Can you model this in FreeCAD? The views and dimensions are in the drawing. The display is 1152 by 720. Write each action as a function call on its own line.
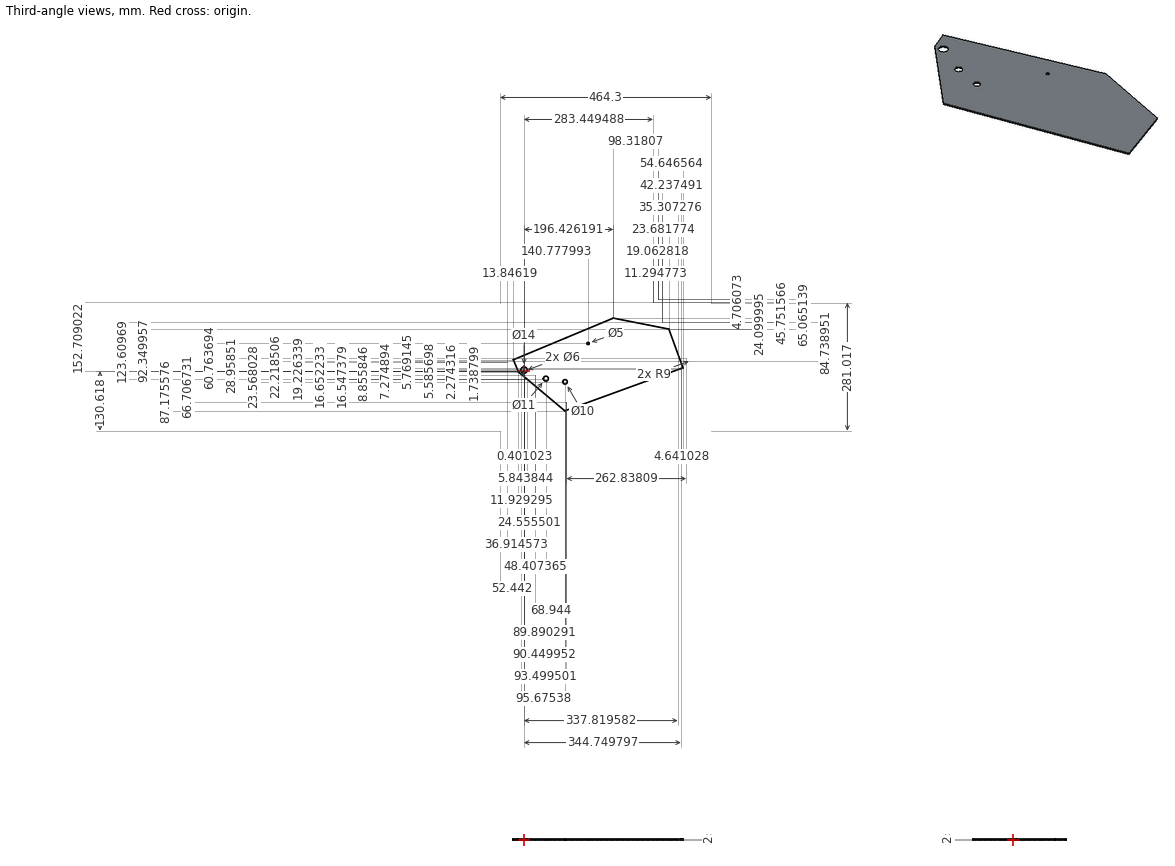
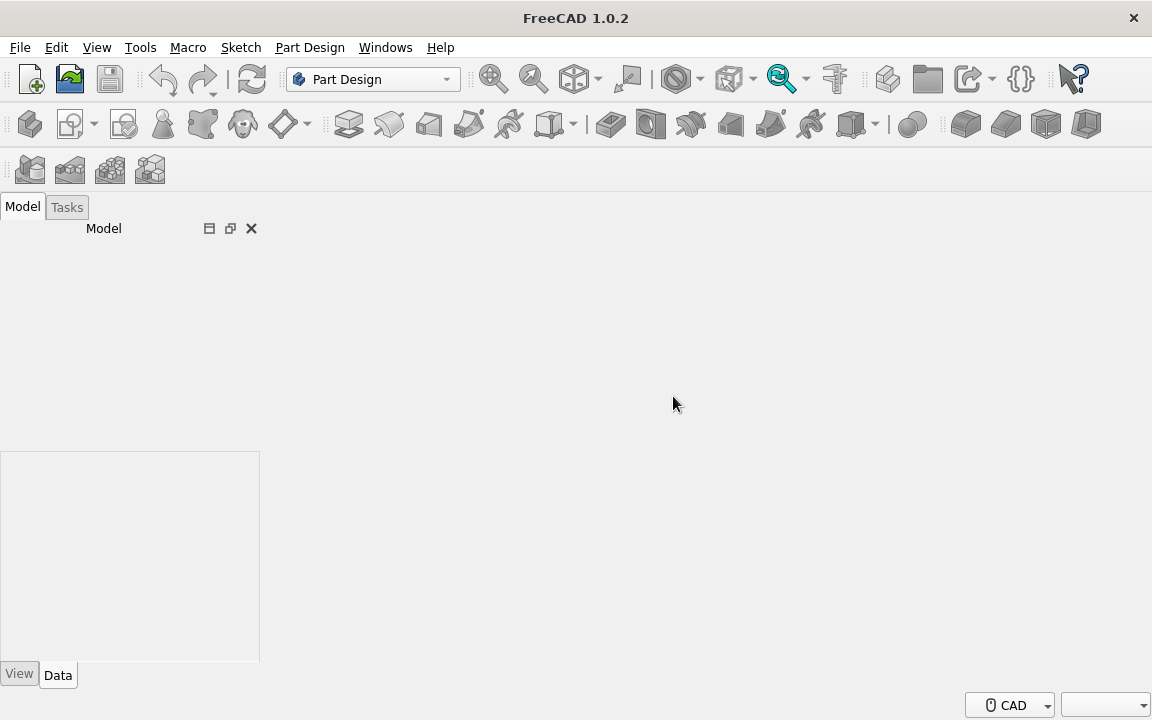
click(30, 80)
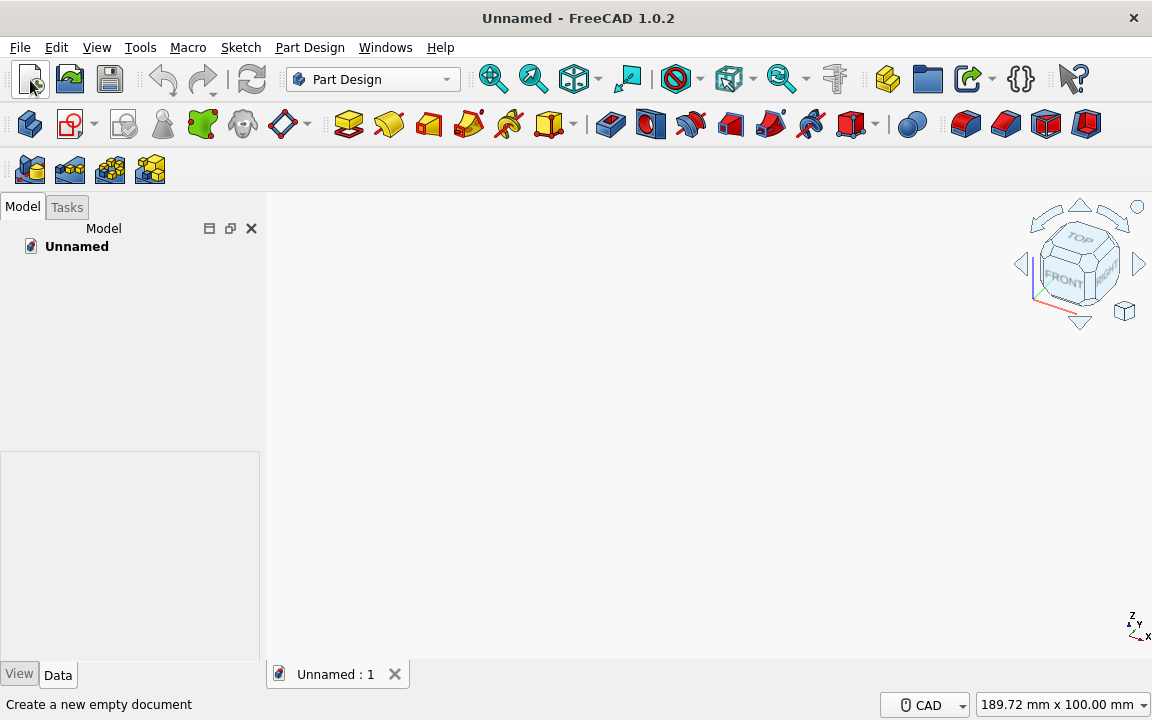
click(70, 124)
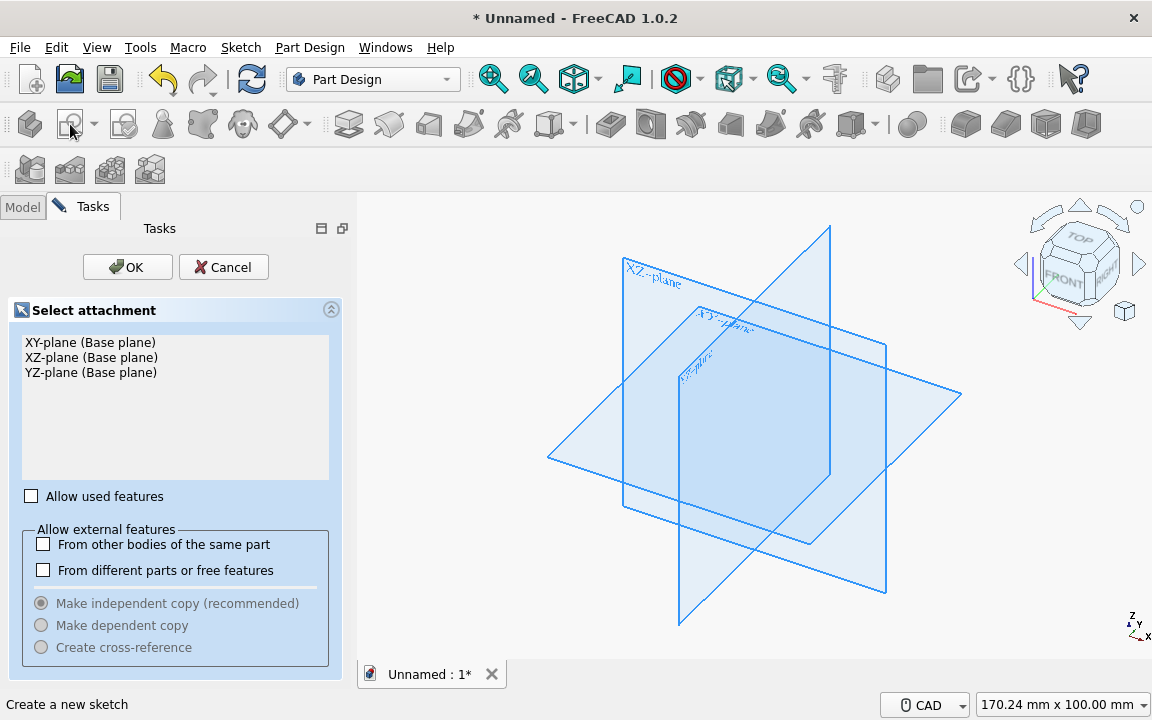
click(82, 342)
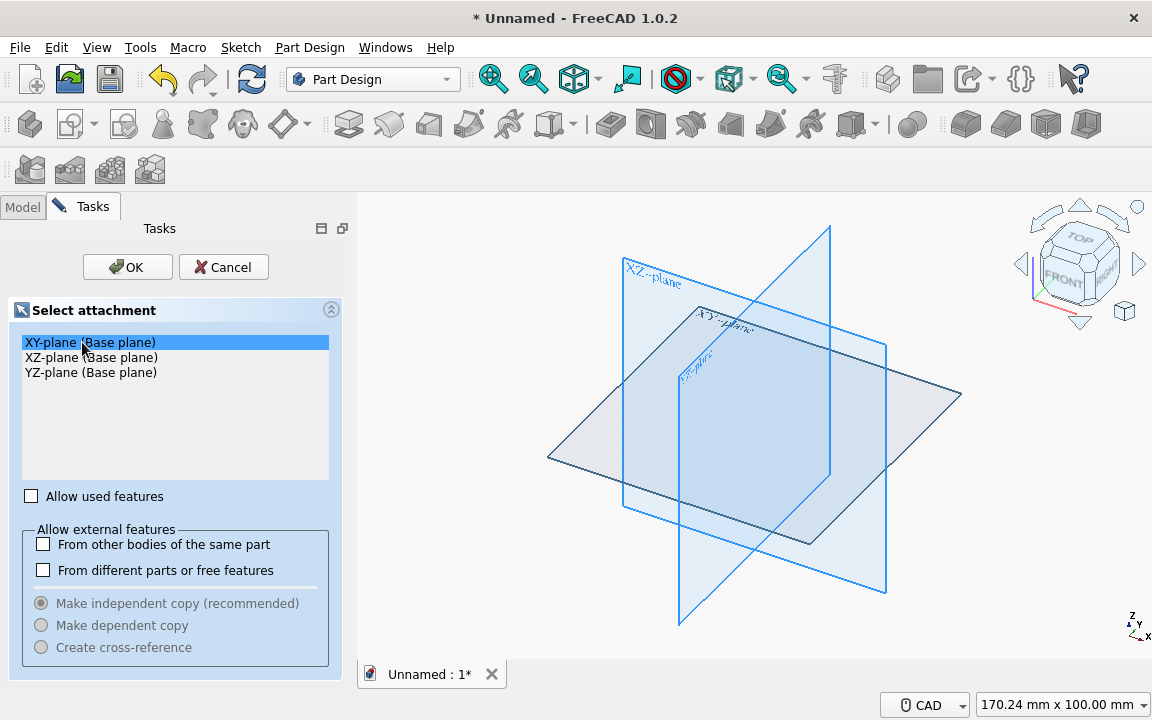
click(128, 267)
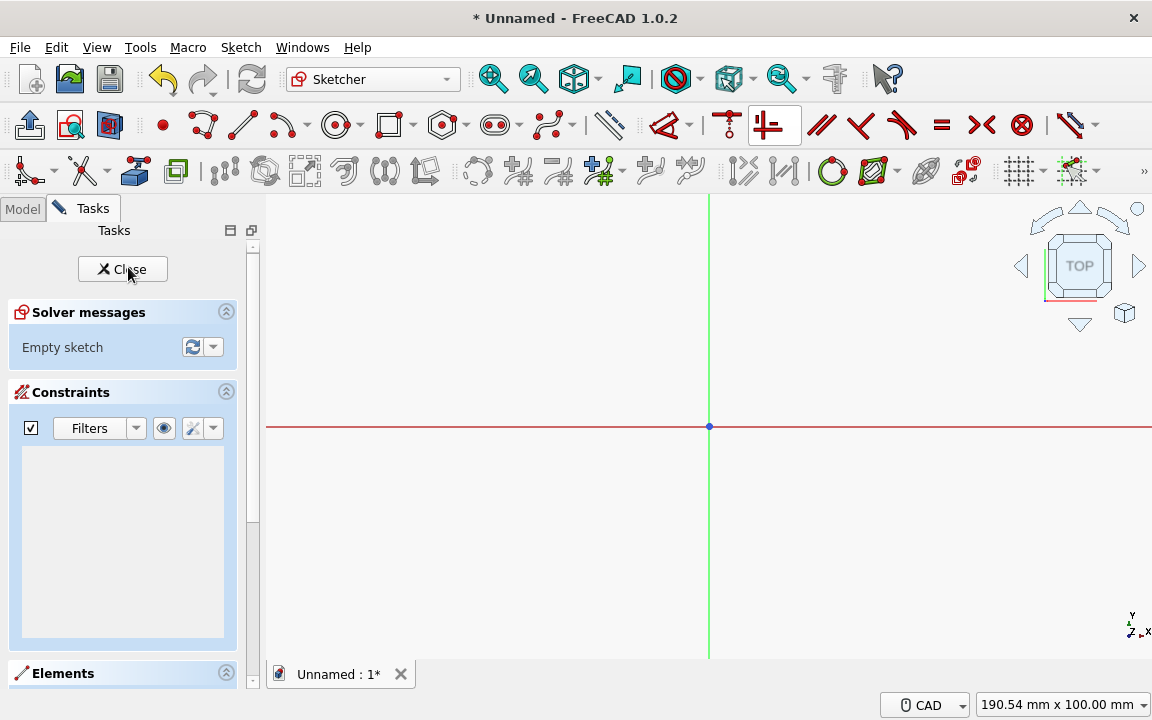
scroll(294, 368, down, 6)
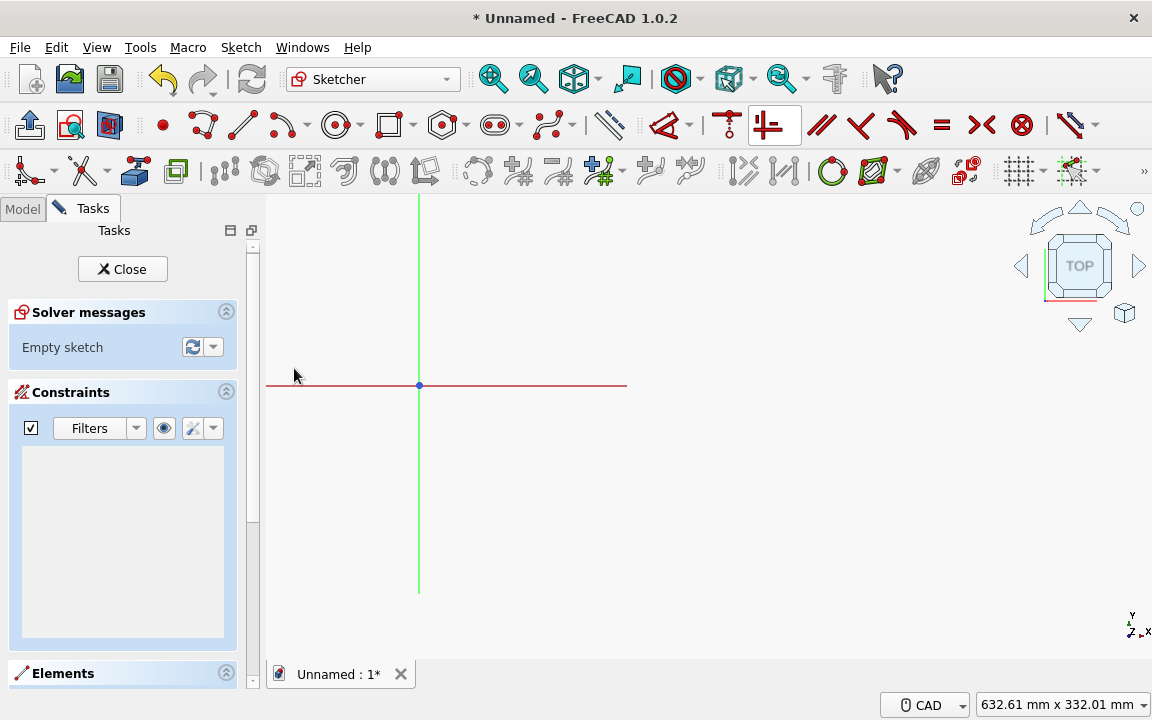
key(g)
key(m)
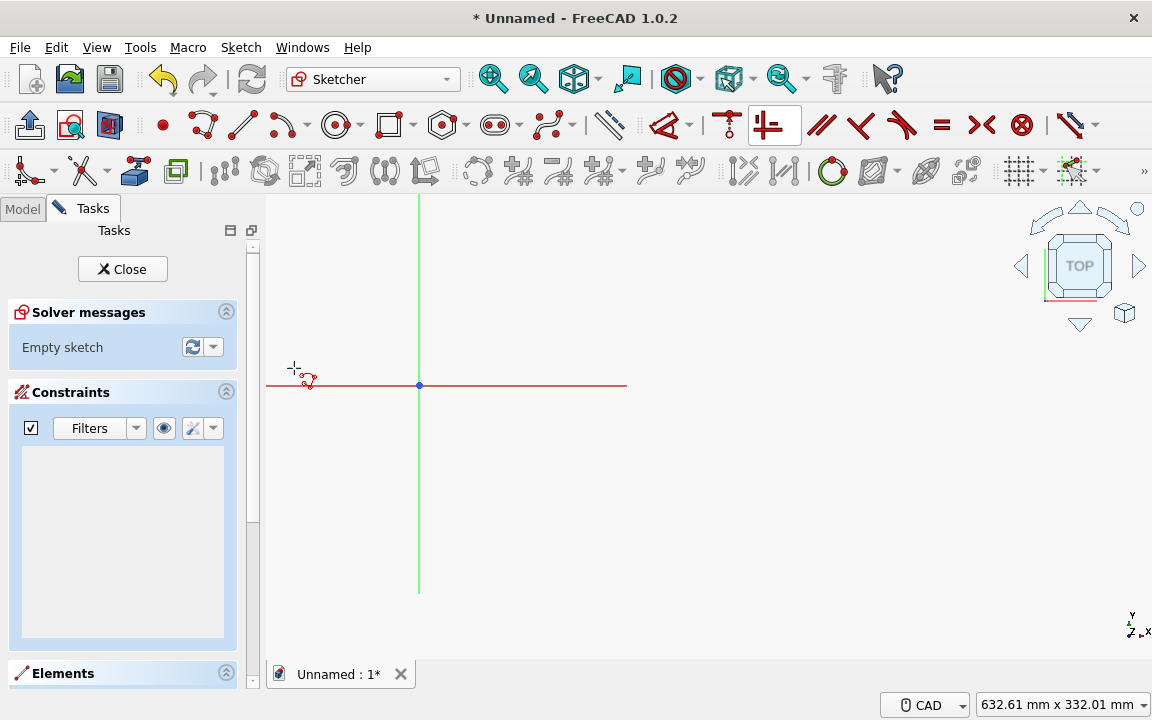
click(918, 345)
click(550, 479)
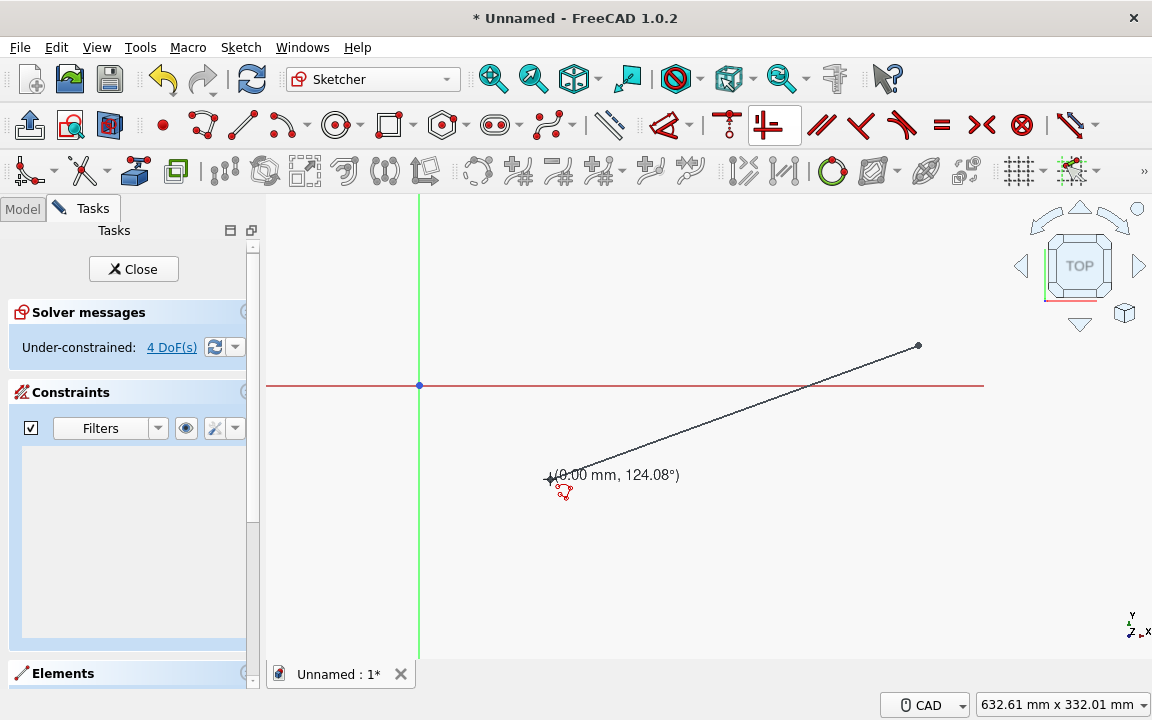
scroll(427, 376, up, 4)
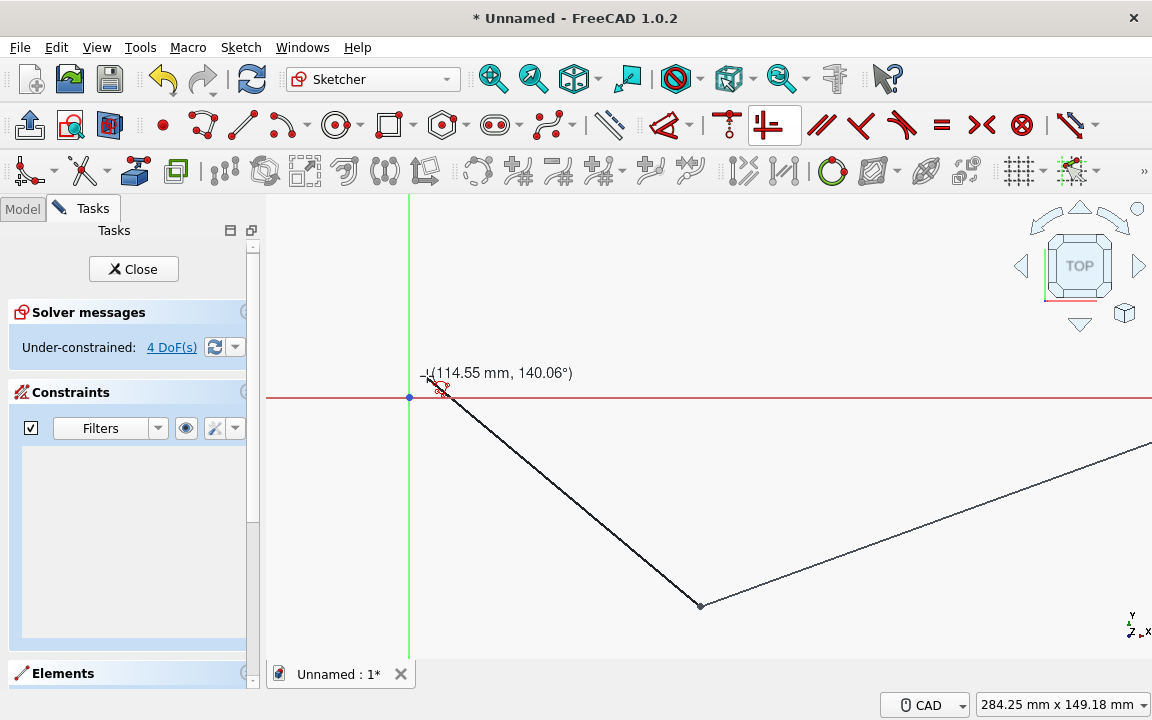
click(427, 376)
right_click(427, 376)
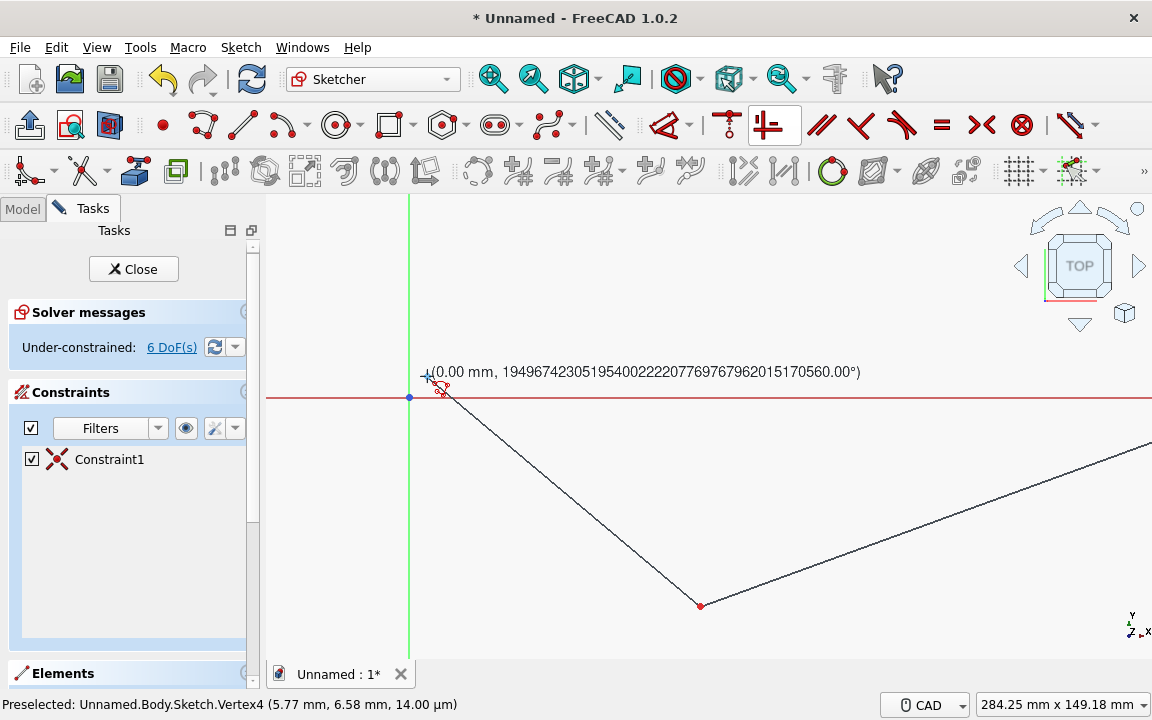
click(391, 419)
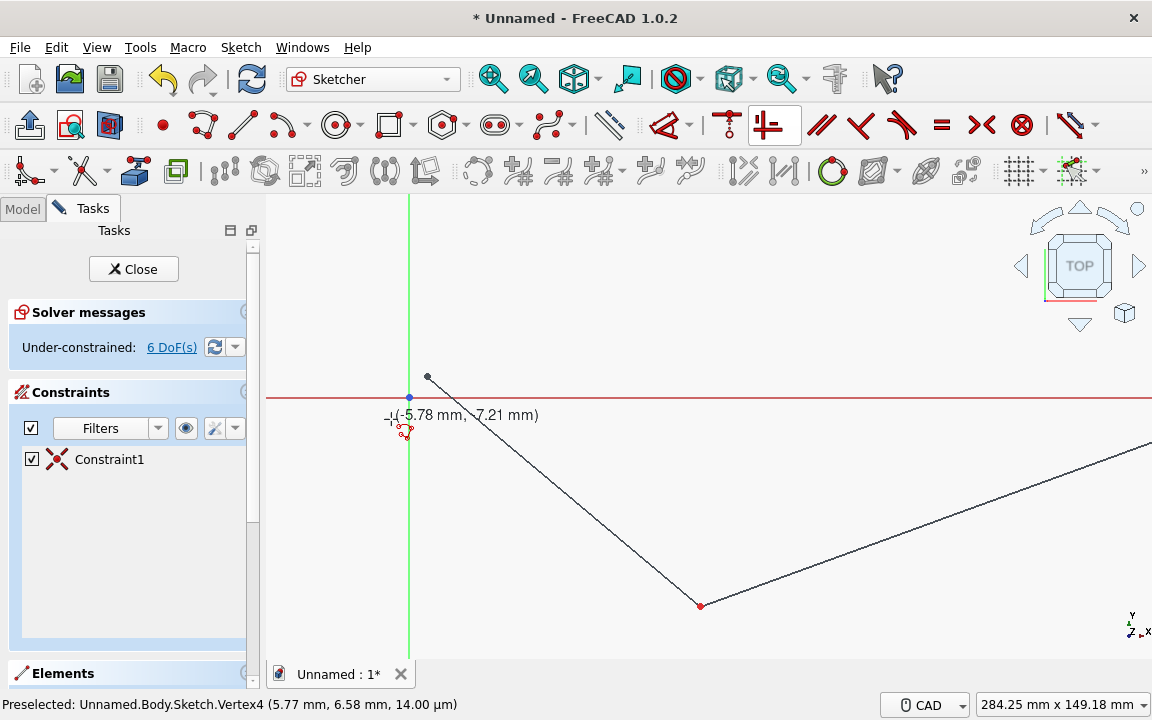
scroll(370, 376, down, 4)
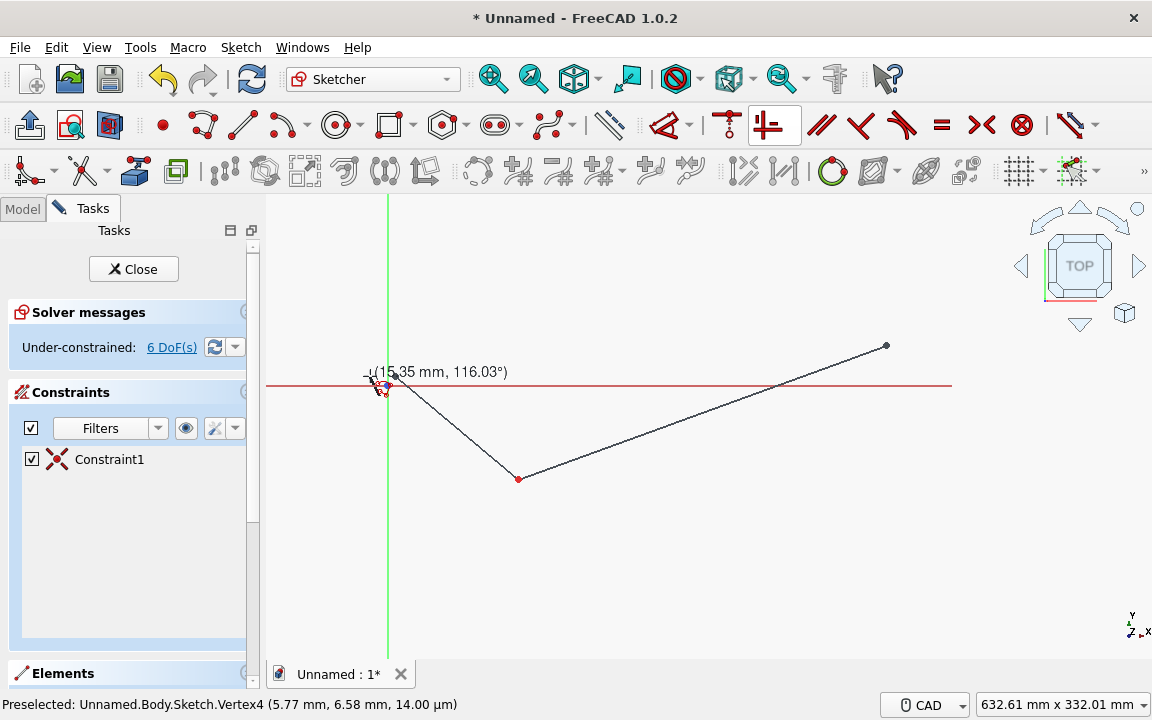
click(513, 508)
click(895, 369)
right_click(895, 369)